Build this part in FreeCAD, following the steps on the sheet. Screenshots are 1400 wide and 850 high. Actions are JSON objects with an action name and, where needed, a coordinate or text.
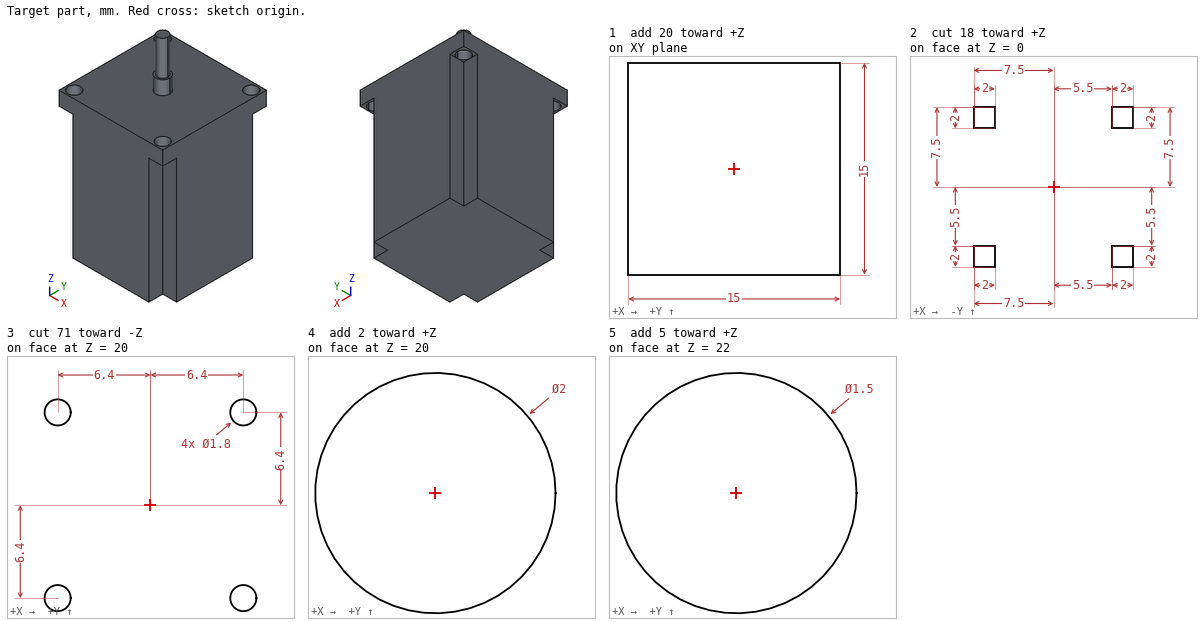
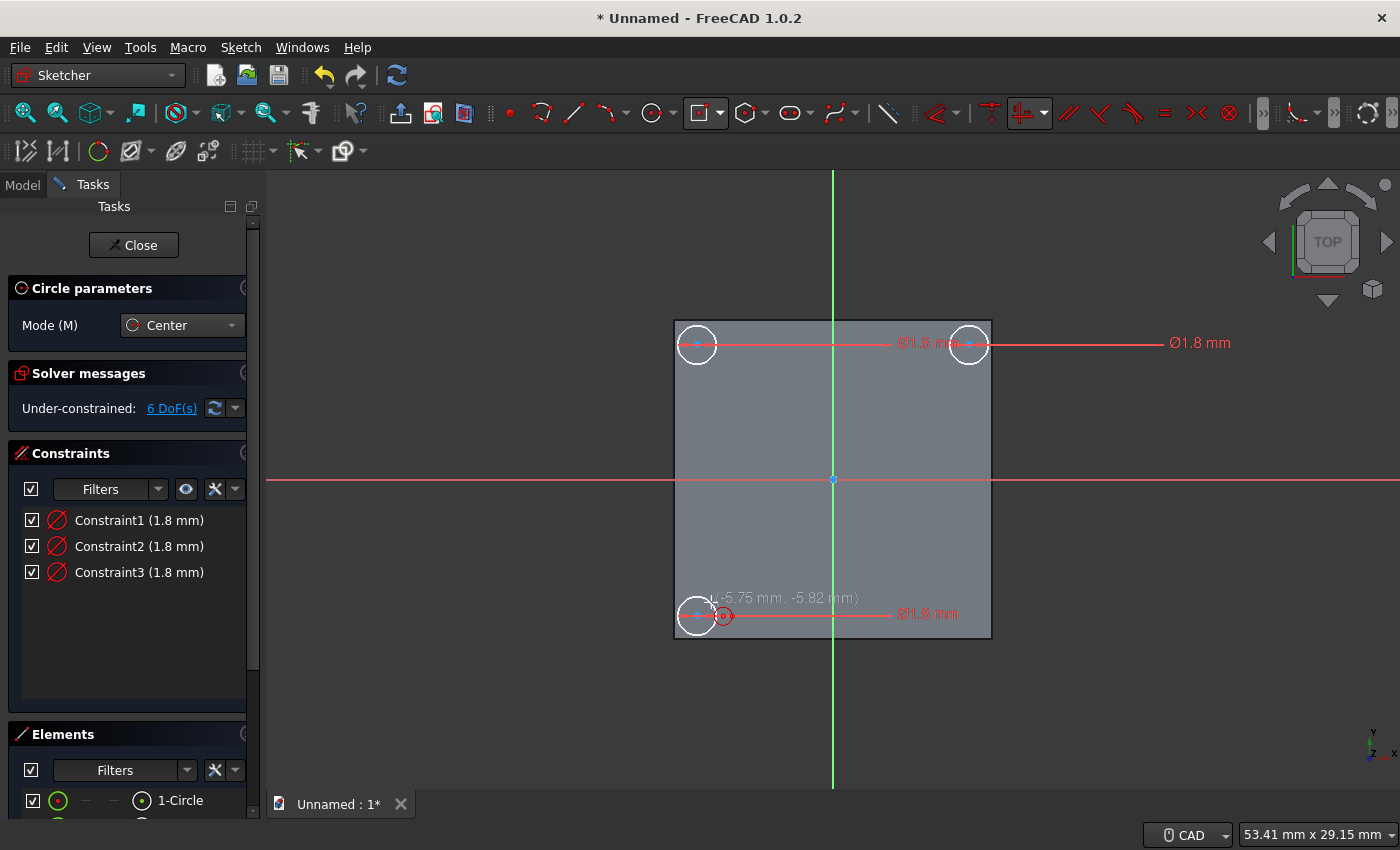
{"action": "left_click", "coordinate": [969, 615]}
{"action": "mouse_move", "coordinate": [982, 602]}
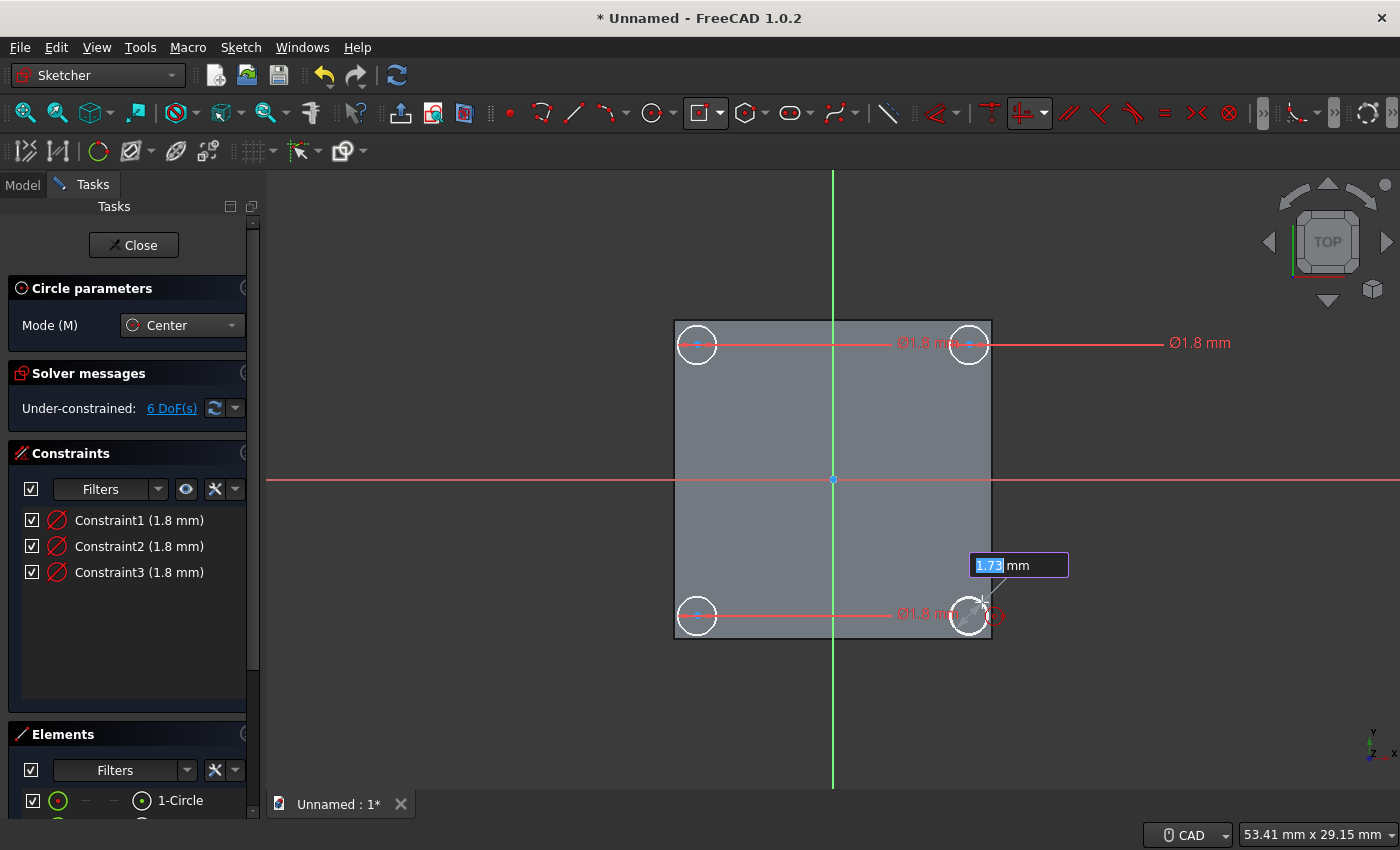
{"action": "type", "text": "1.8"}
{"action": "key", "text": "Return"}
{"action": "key", "text": "Escape"}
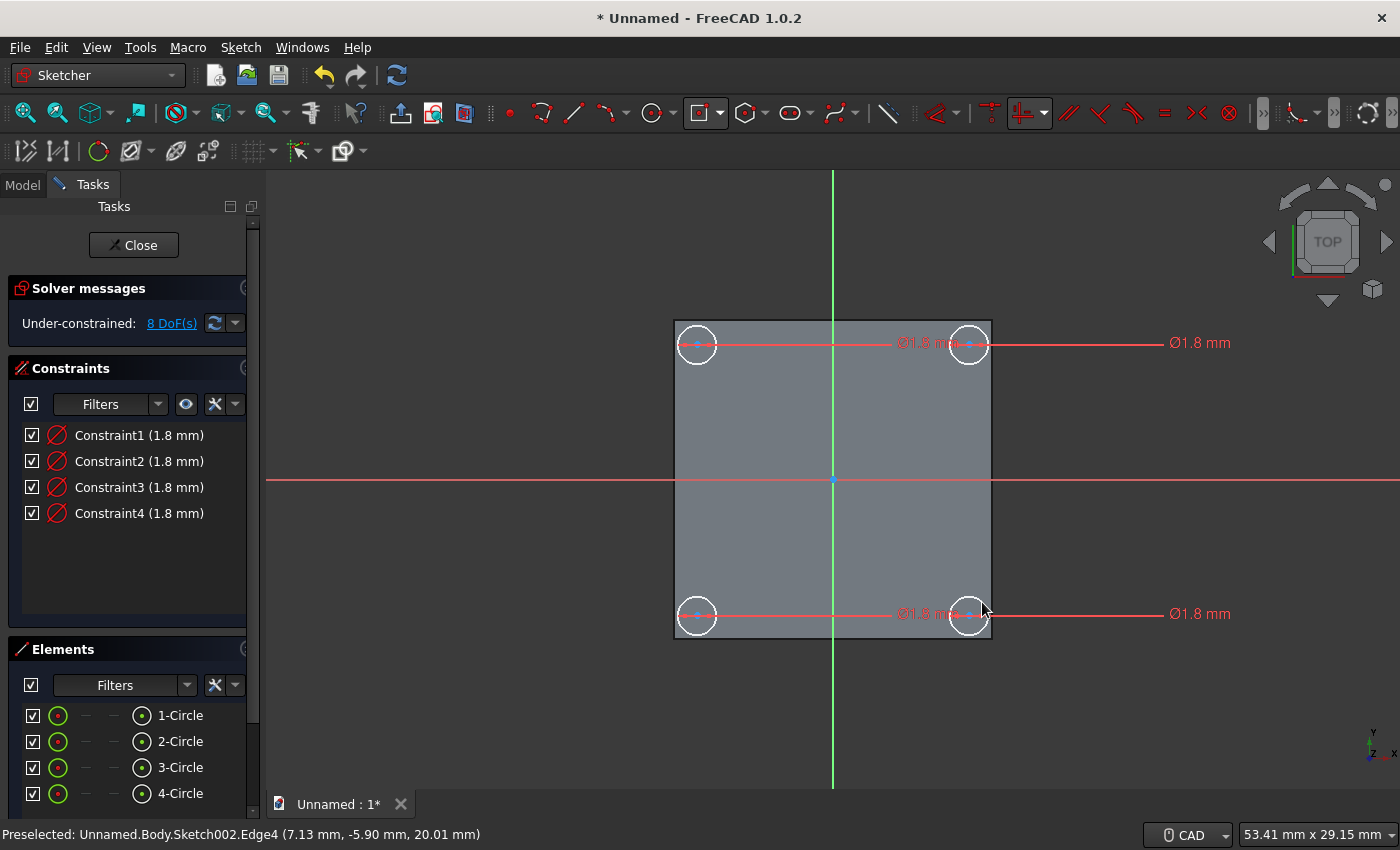
{"action": "left_click", "coordinate": [969, 345]}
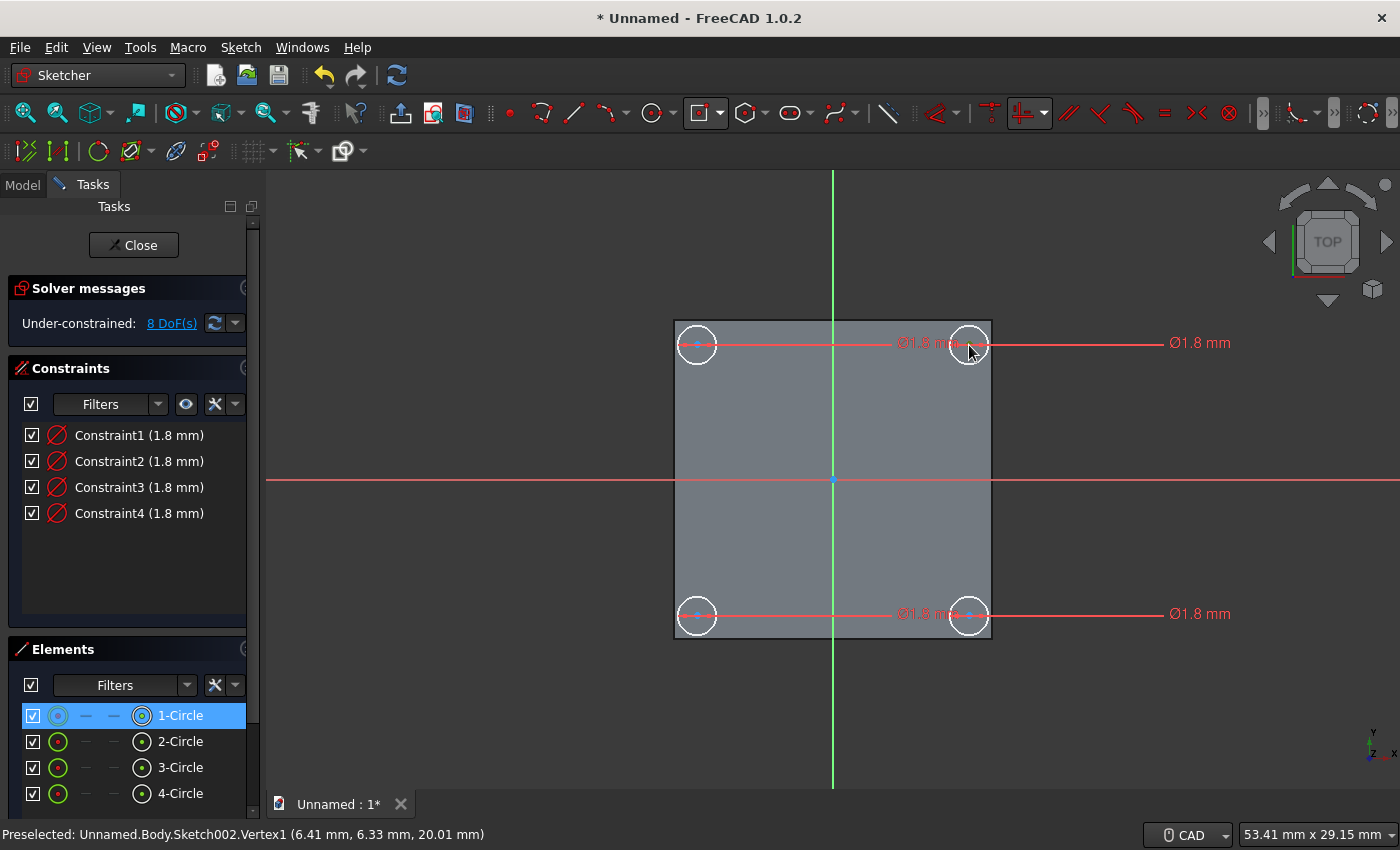
{"action": "left_click", "coordinate": [697, 345]}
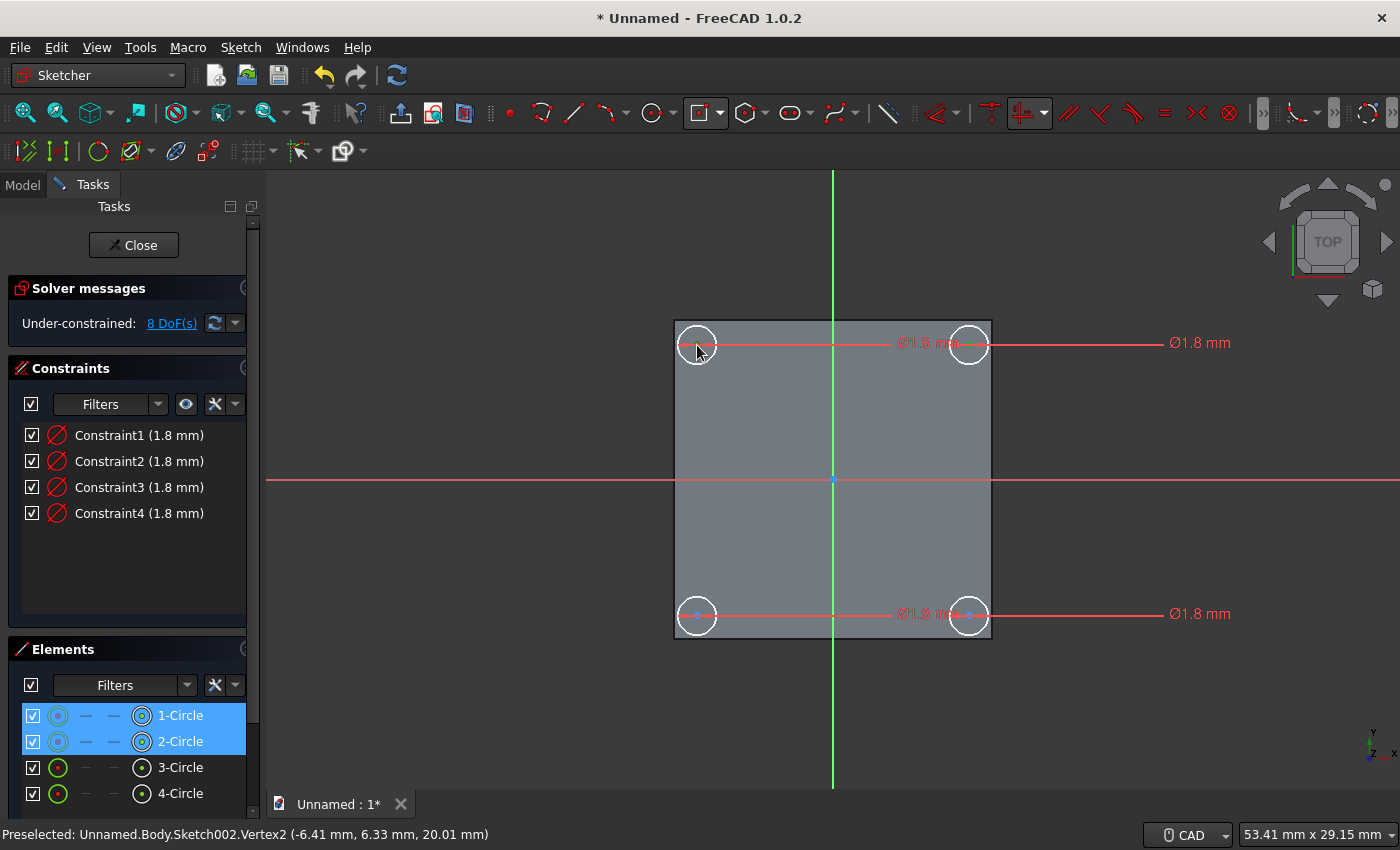
{"action": "left_click", "coordinate": [1046, 114]}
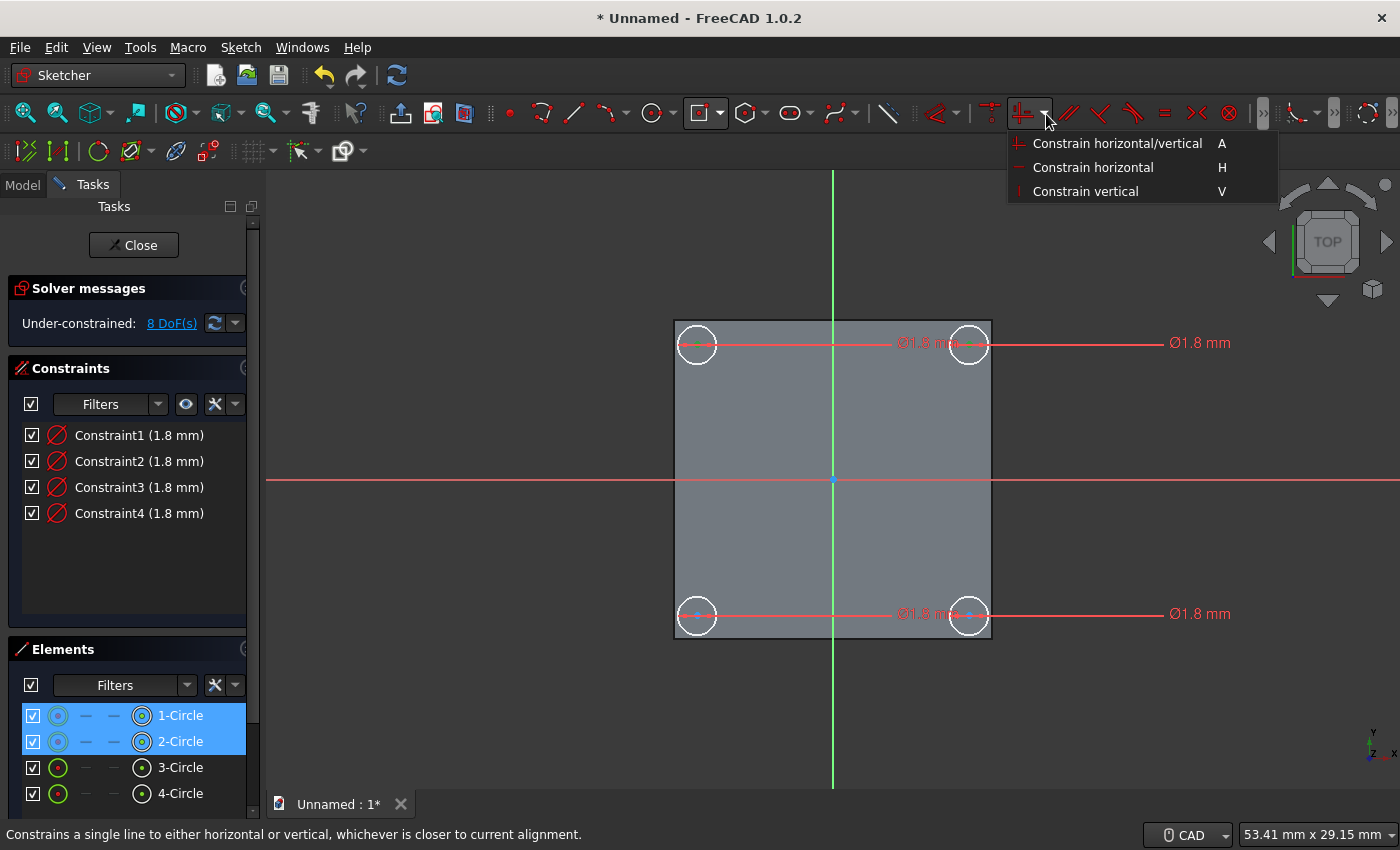
{"action": "left_click", "coordinate": [1143, 167]}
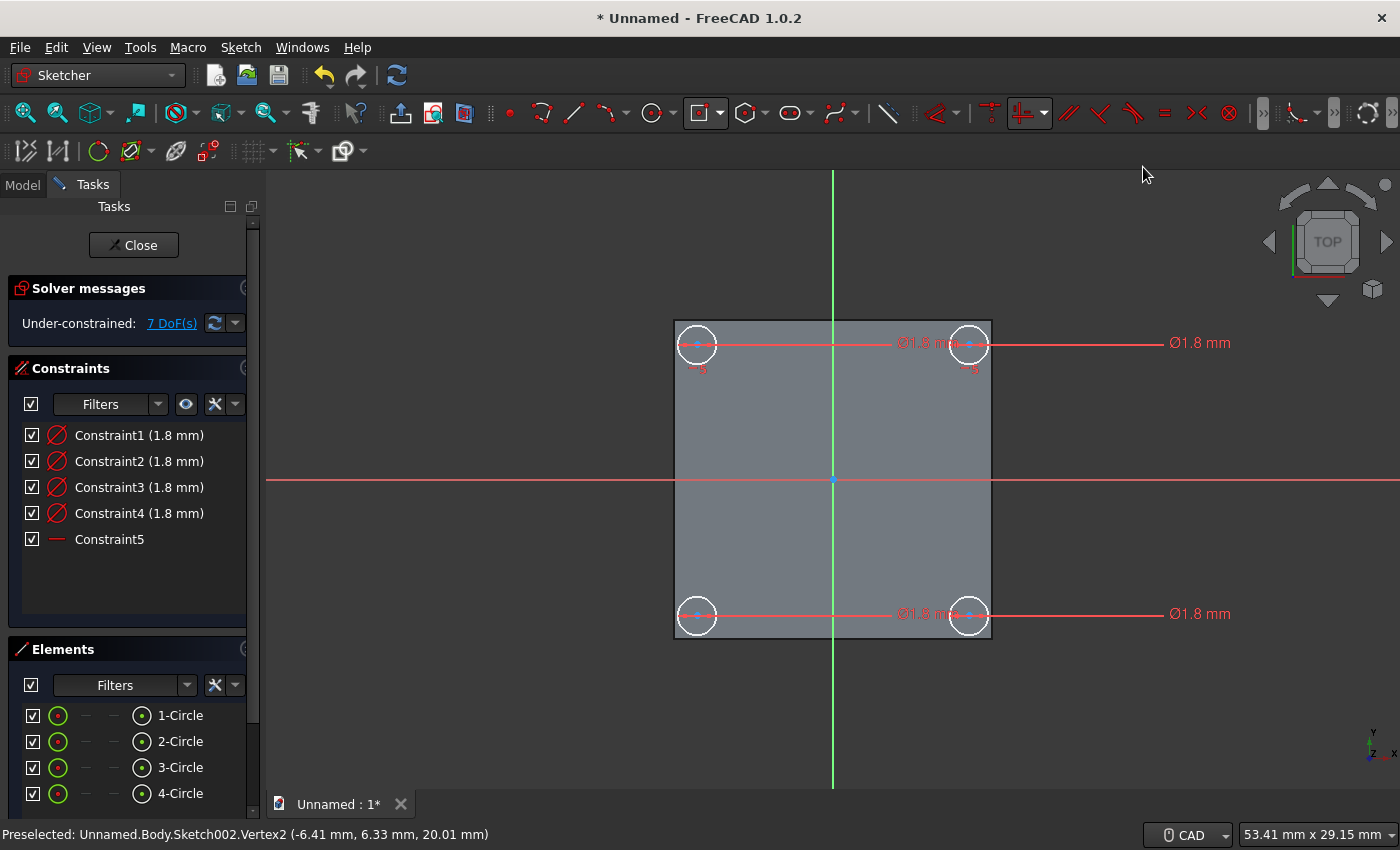
{"action": "left_click", "coordinate": [697, 345]}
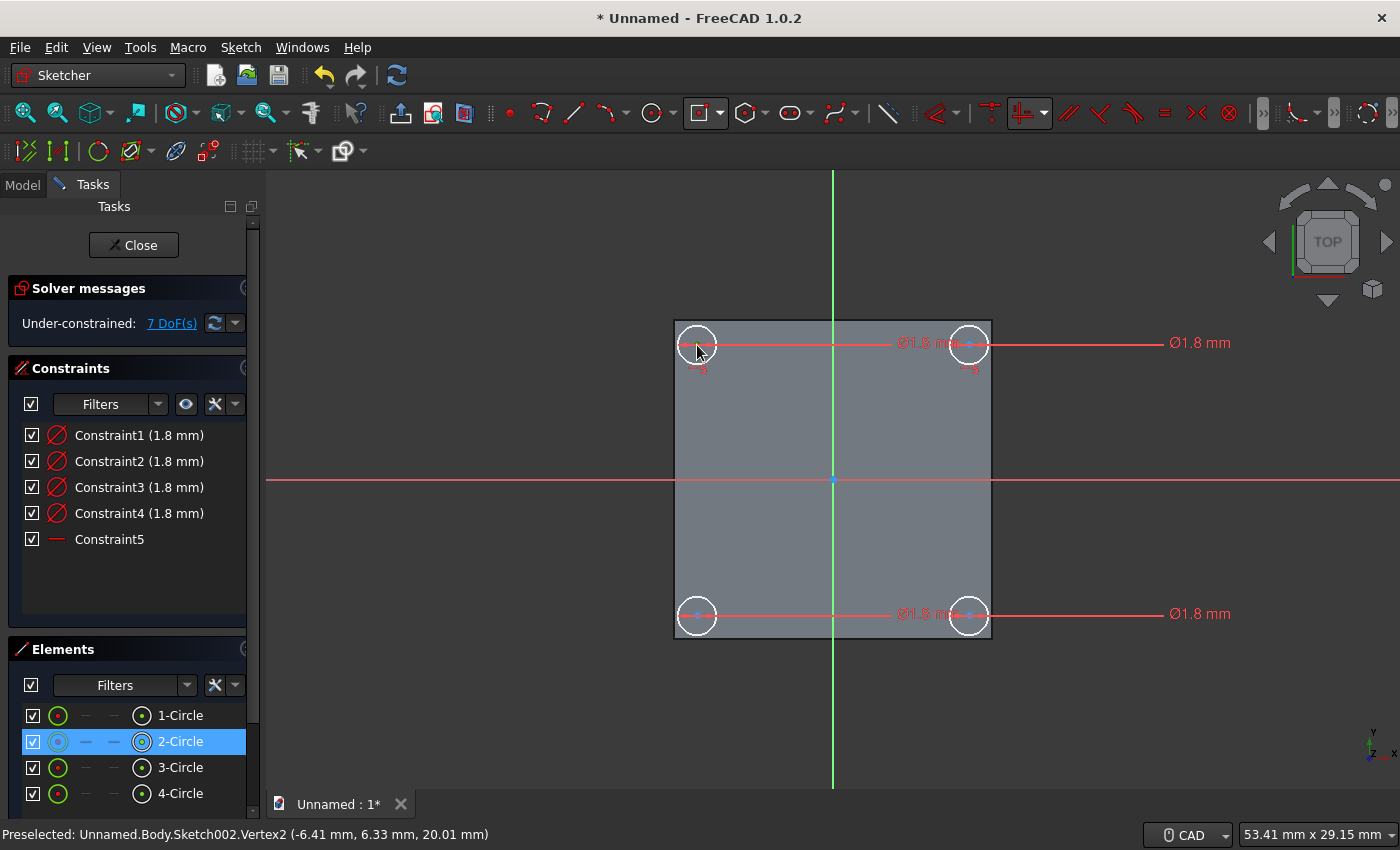
{"action": "left_click", "coordinate": [697, 616]}